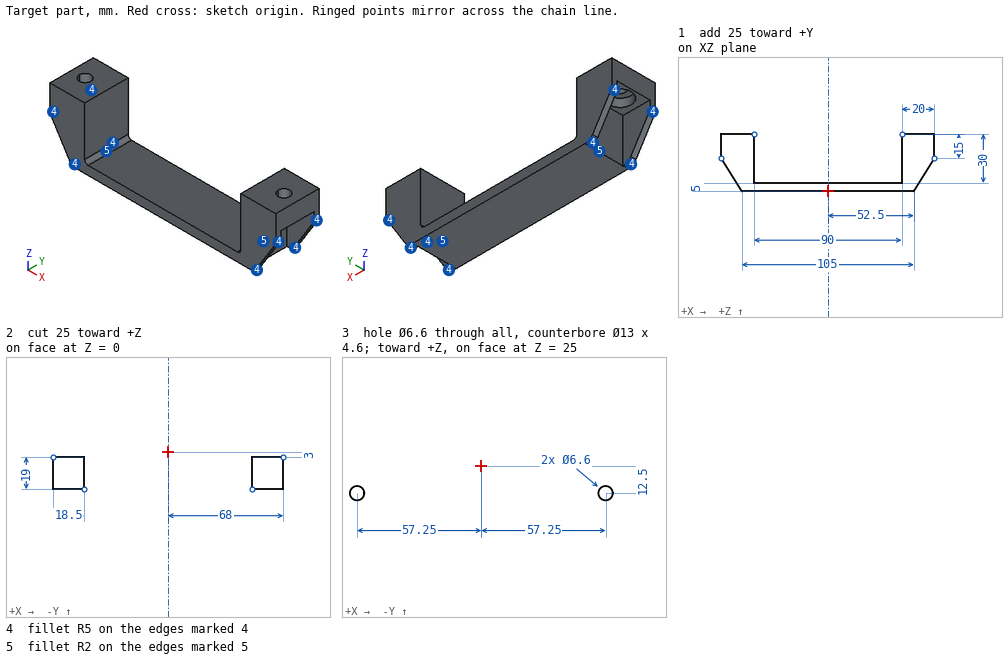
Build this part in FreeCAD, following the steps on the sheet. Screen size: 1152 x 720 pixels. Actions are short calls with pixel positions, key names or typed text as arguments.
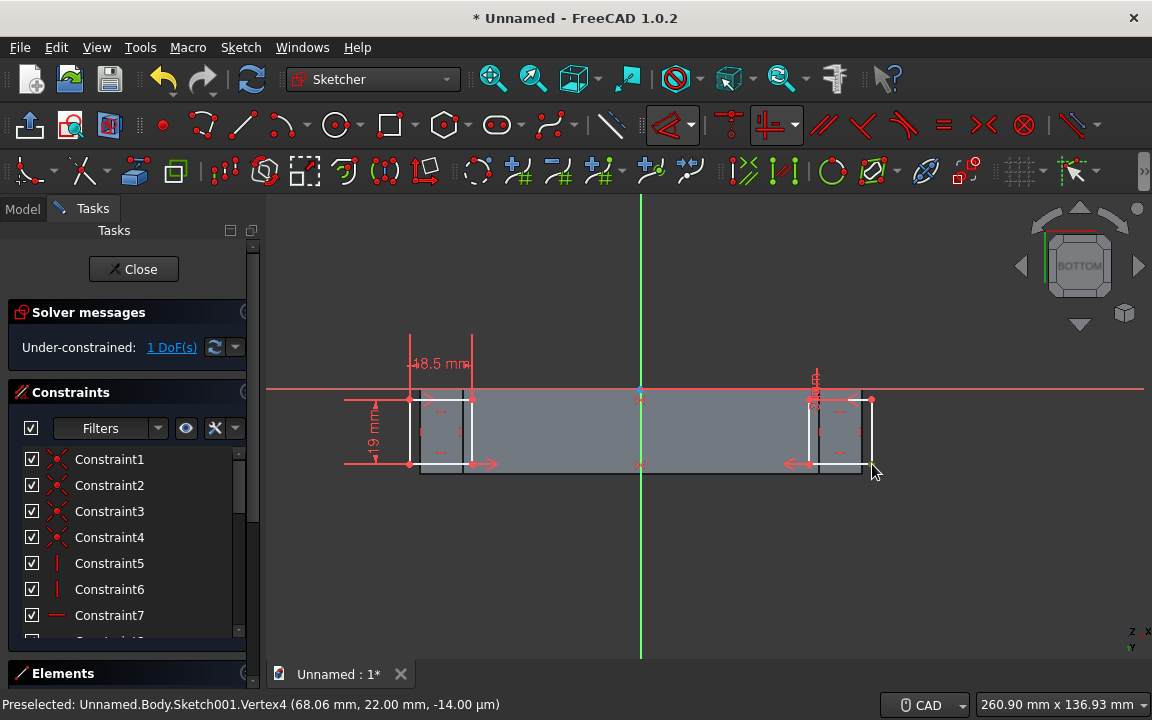
key(l)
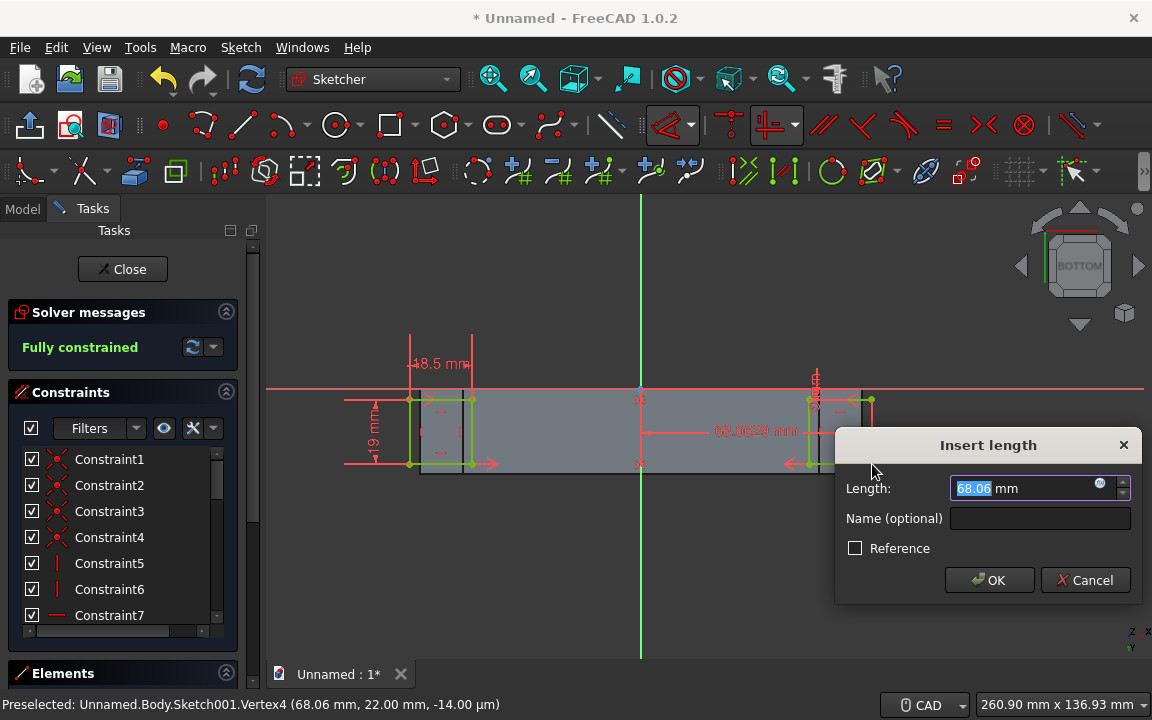
text(68)
key(Return)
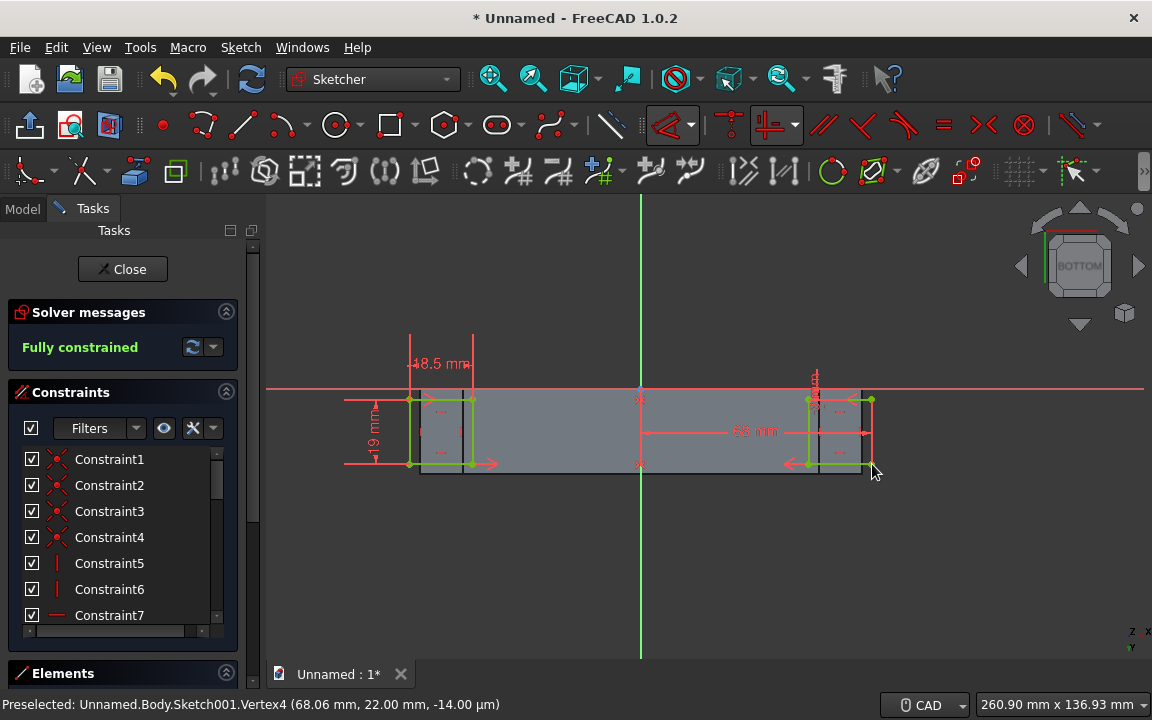
click(123, 269)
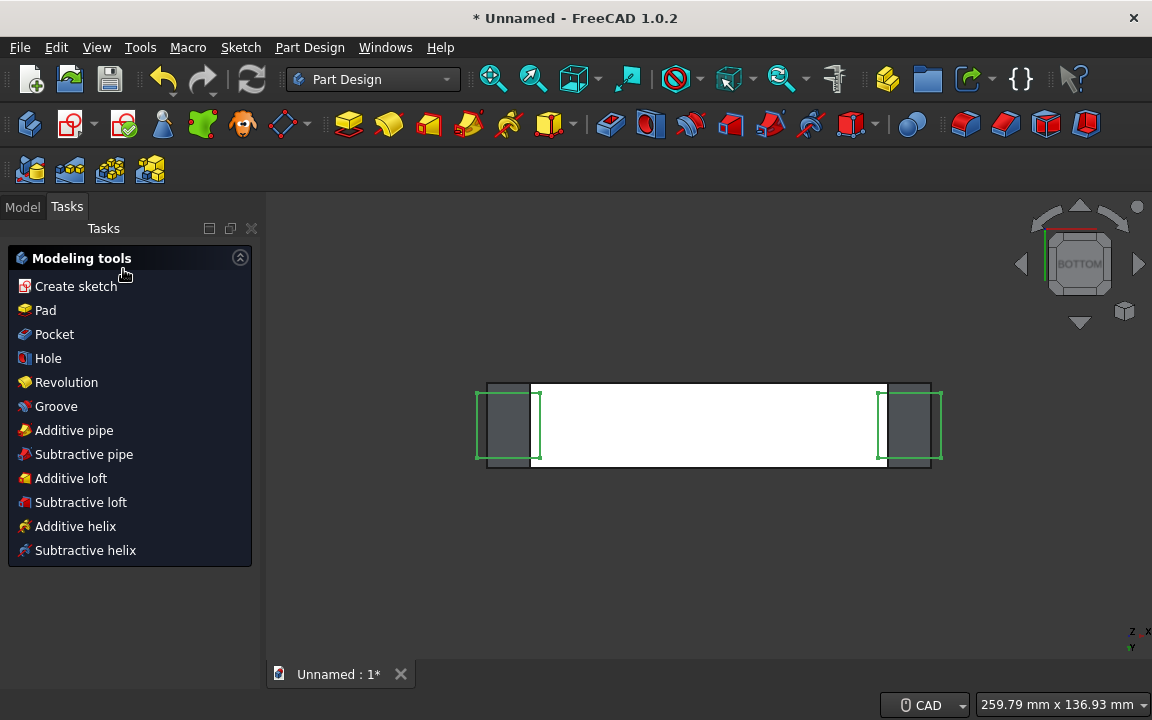
click(612, 124)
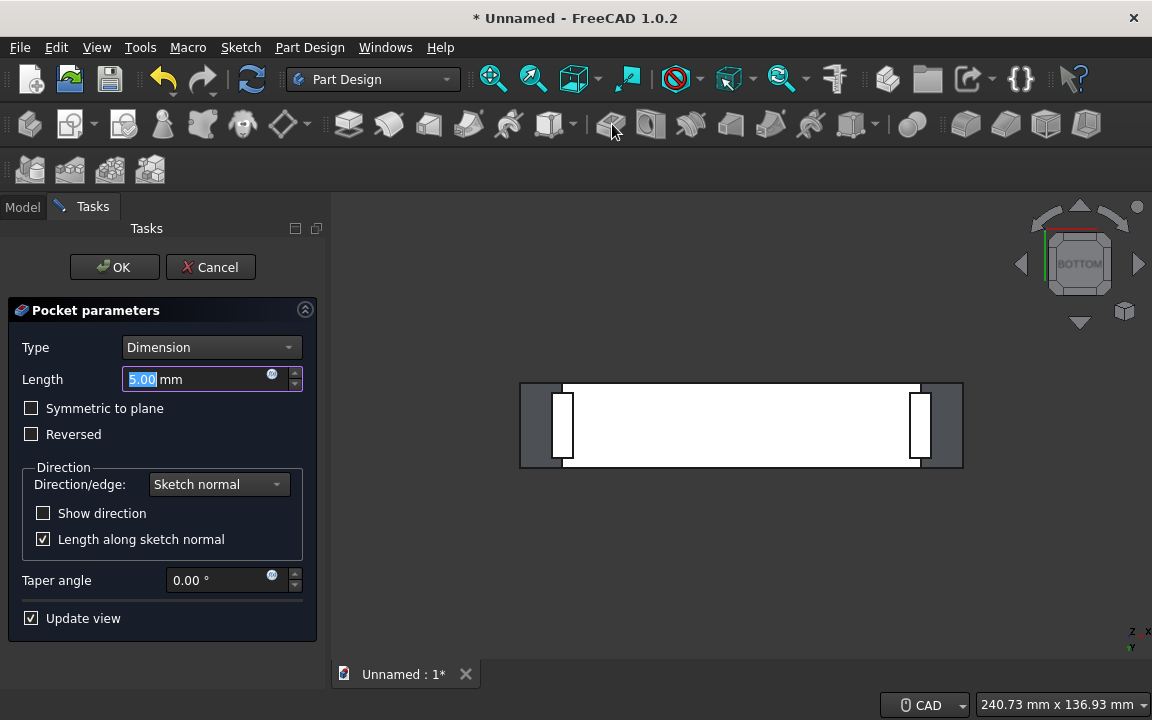
text(25)
key(Tab)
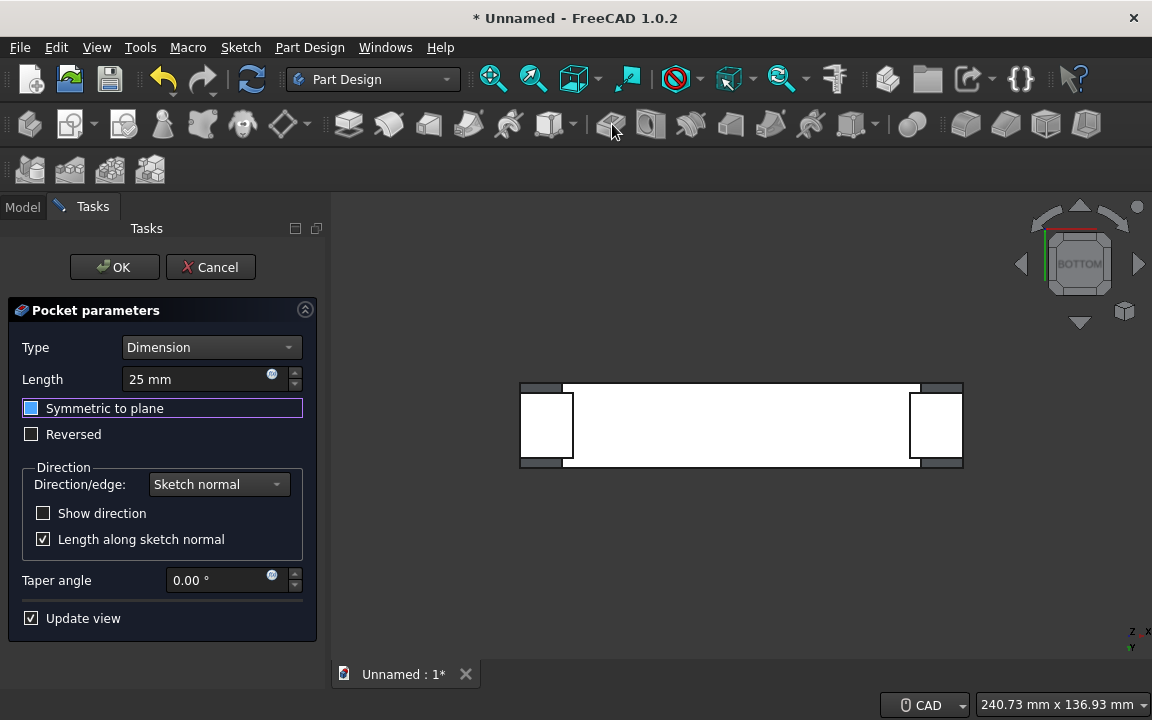
click(115, 267)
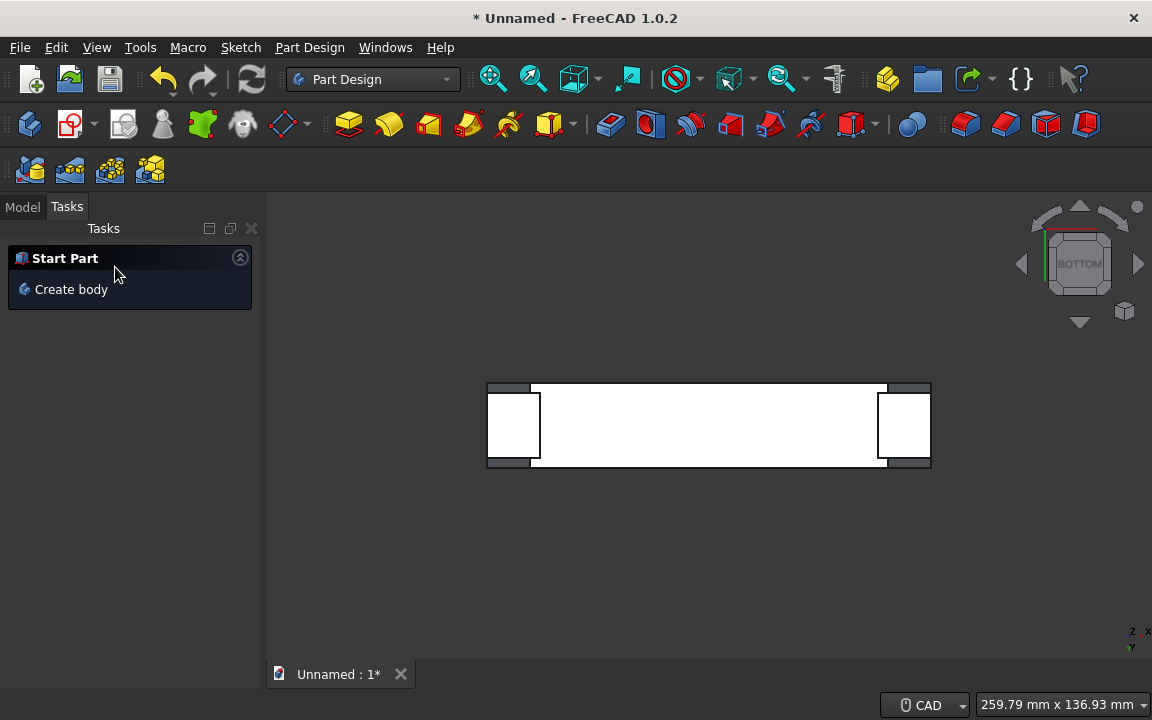
click(514, 425)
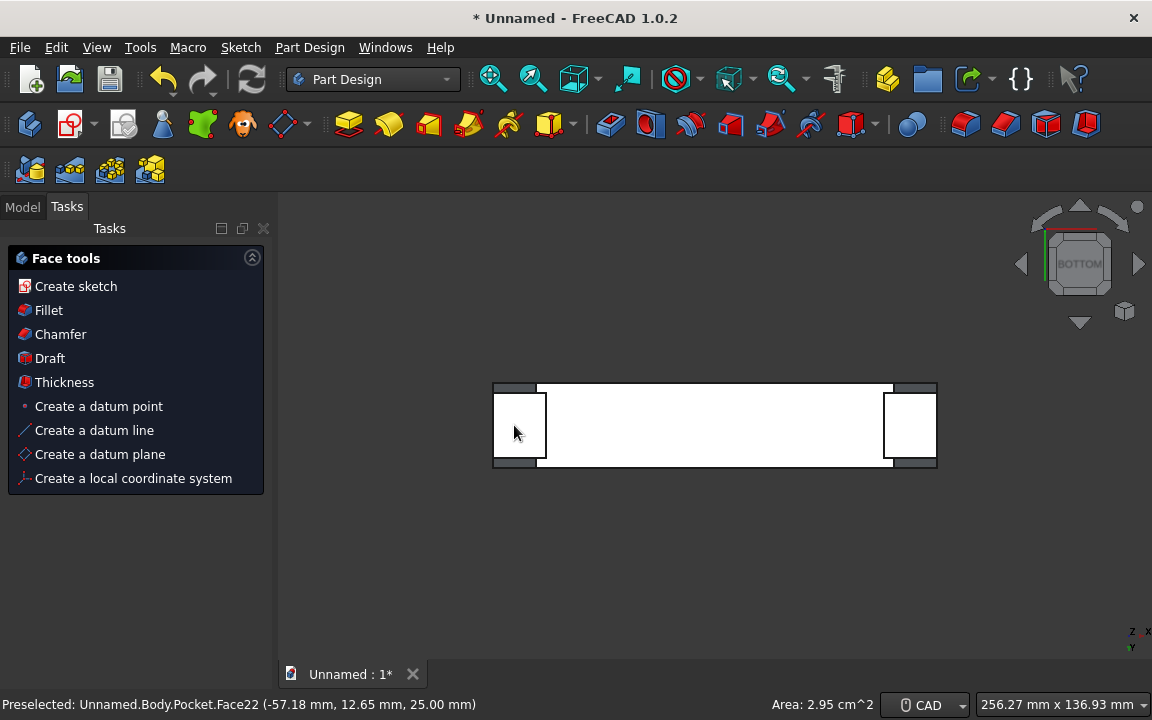
click(70, 124)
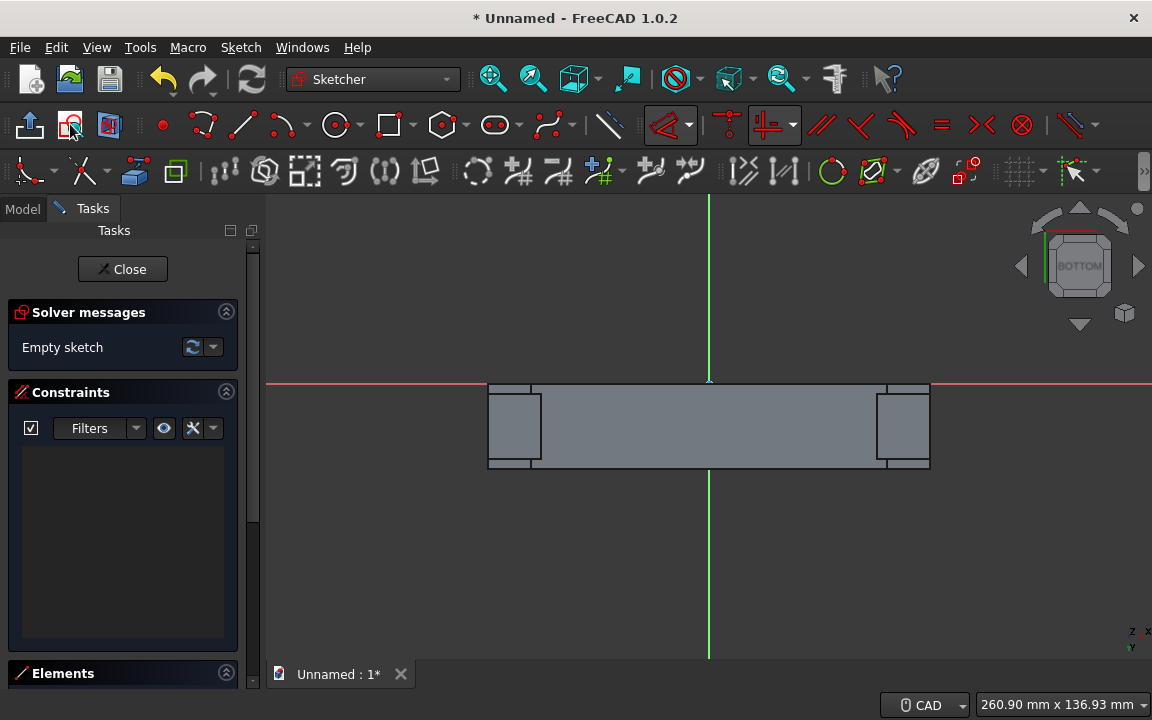
click(110, 126)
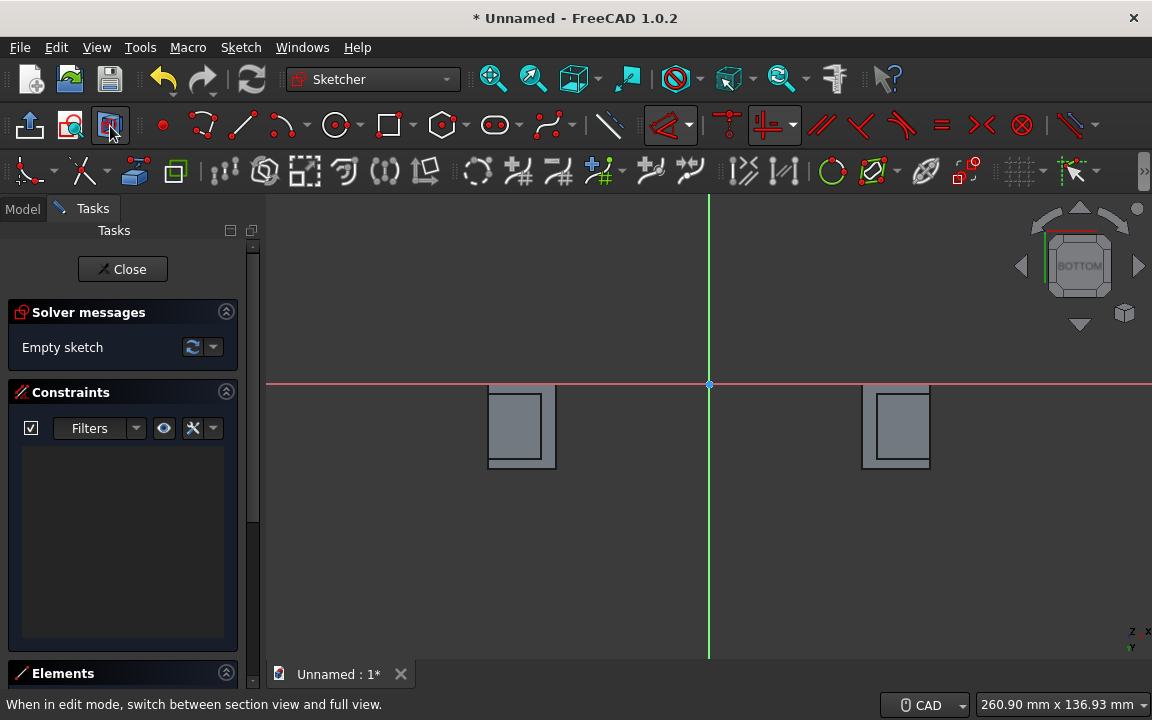
click(336, 126)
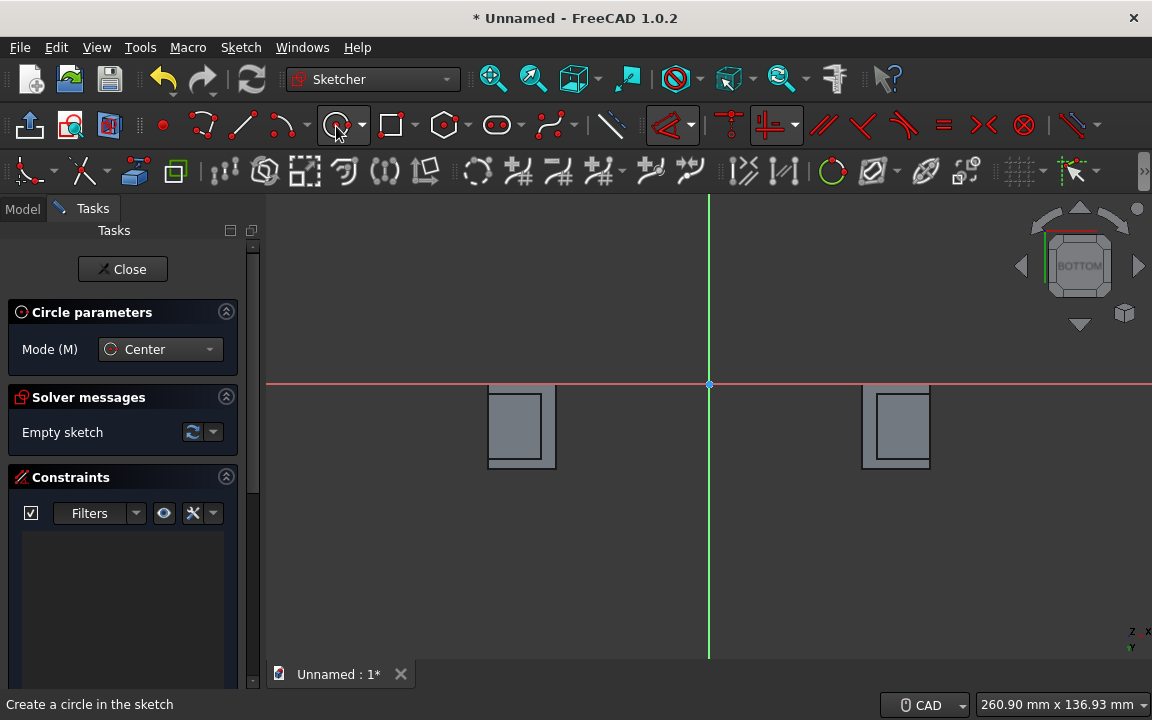
scroll(903, 427, up, 4)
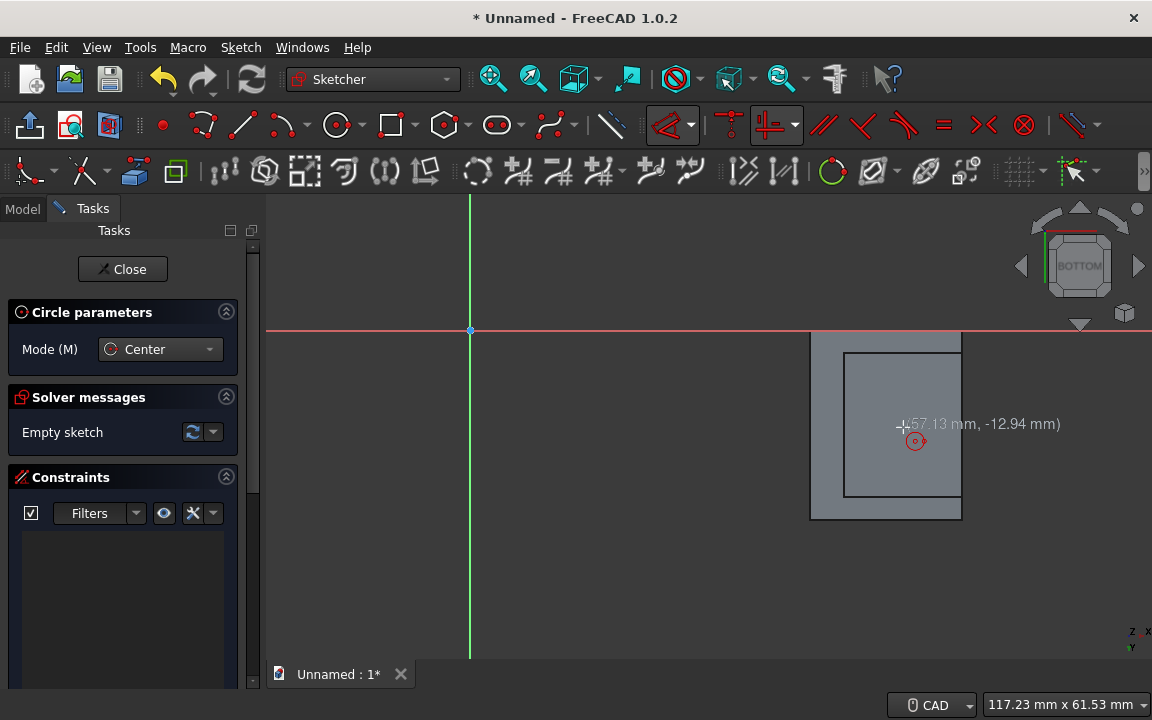
click(903, 425)
move(921, 408)